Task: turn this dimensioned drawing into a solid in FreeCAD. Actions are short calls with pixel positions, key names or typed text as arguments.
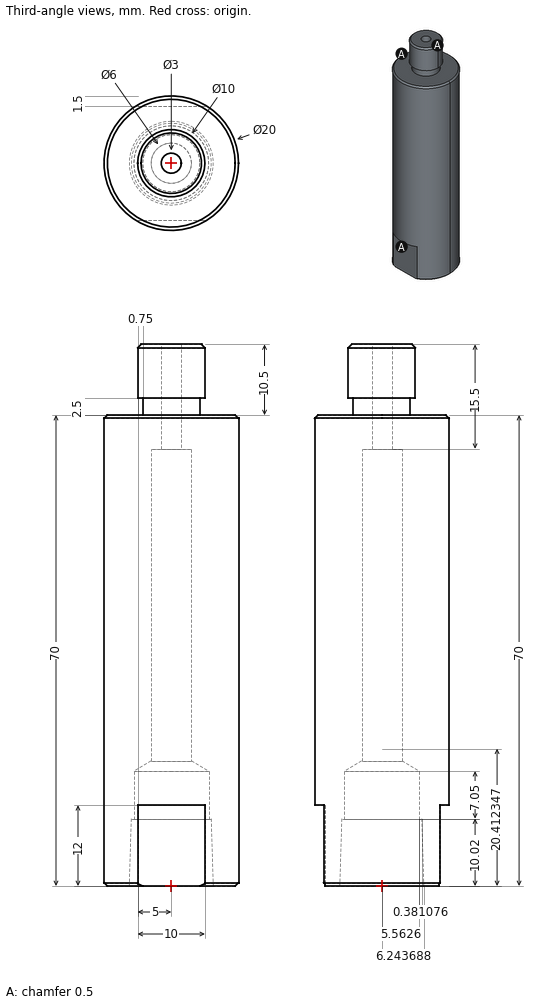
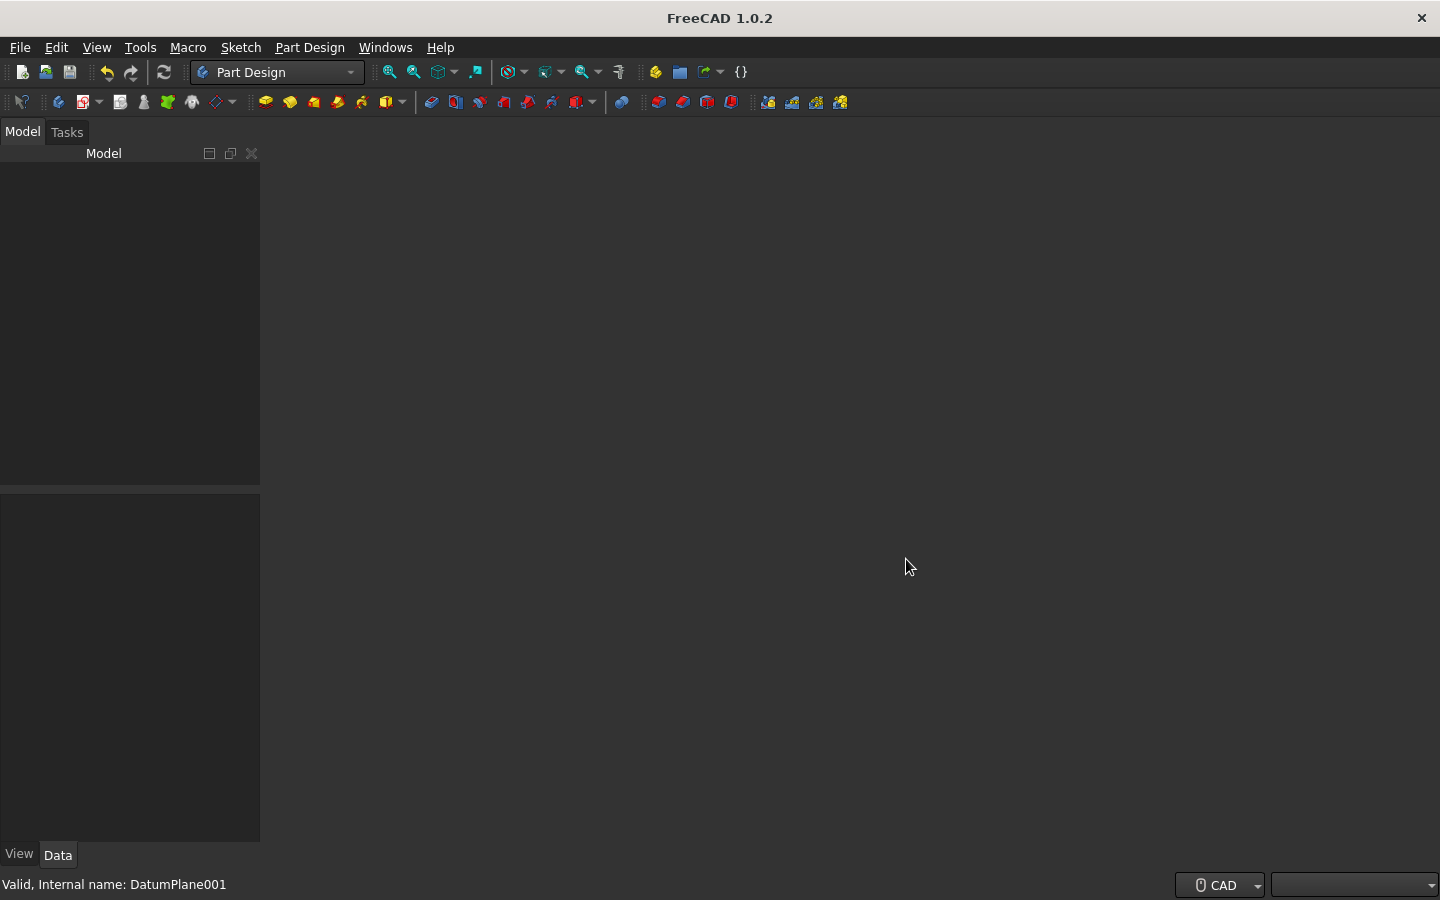
click(22, 72)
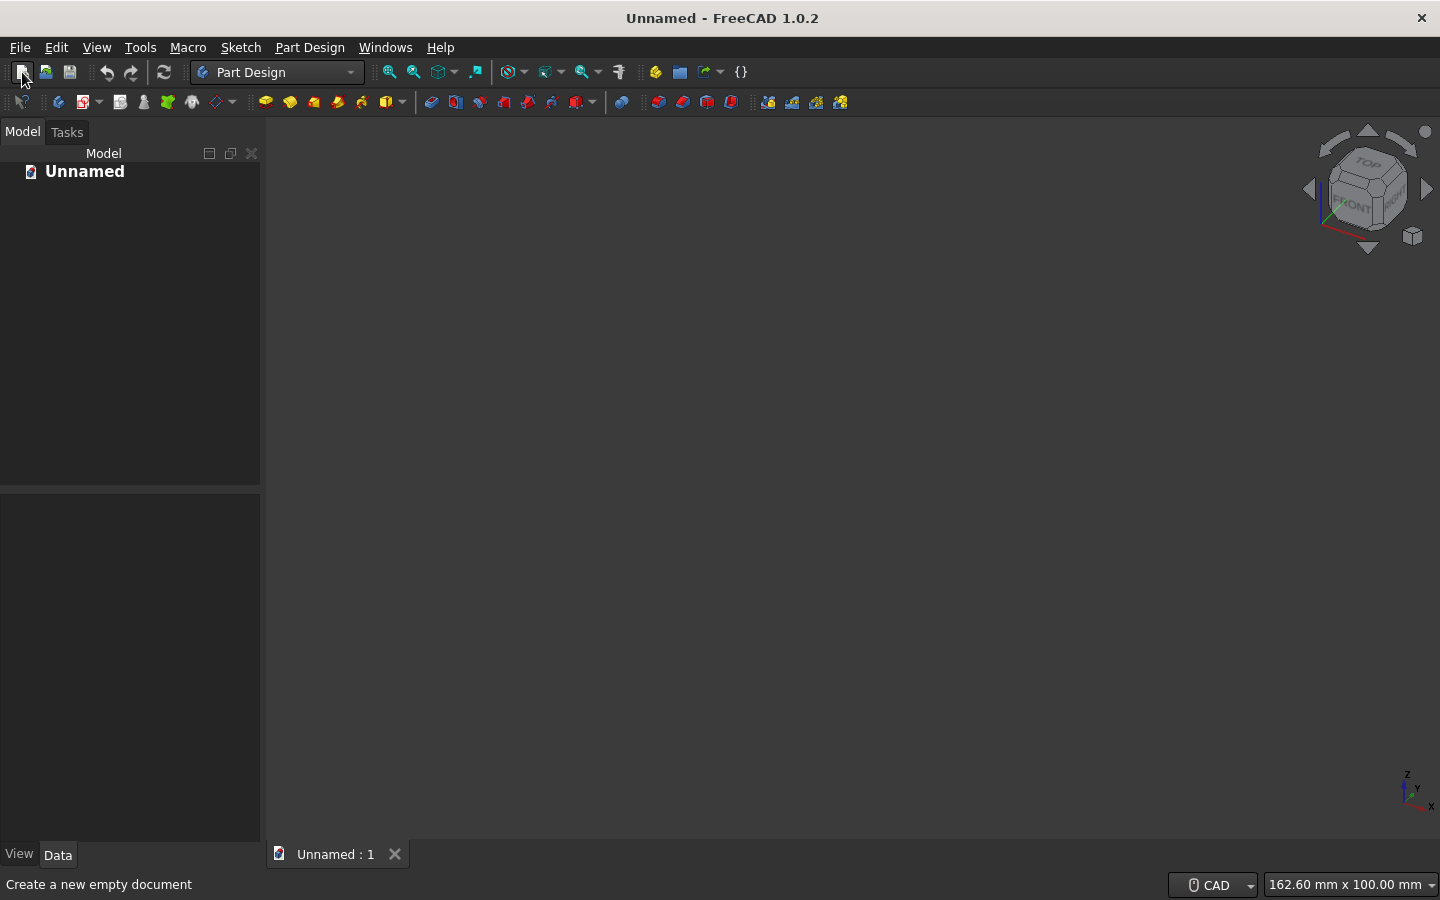
click(84, 102)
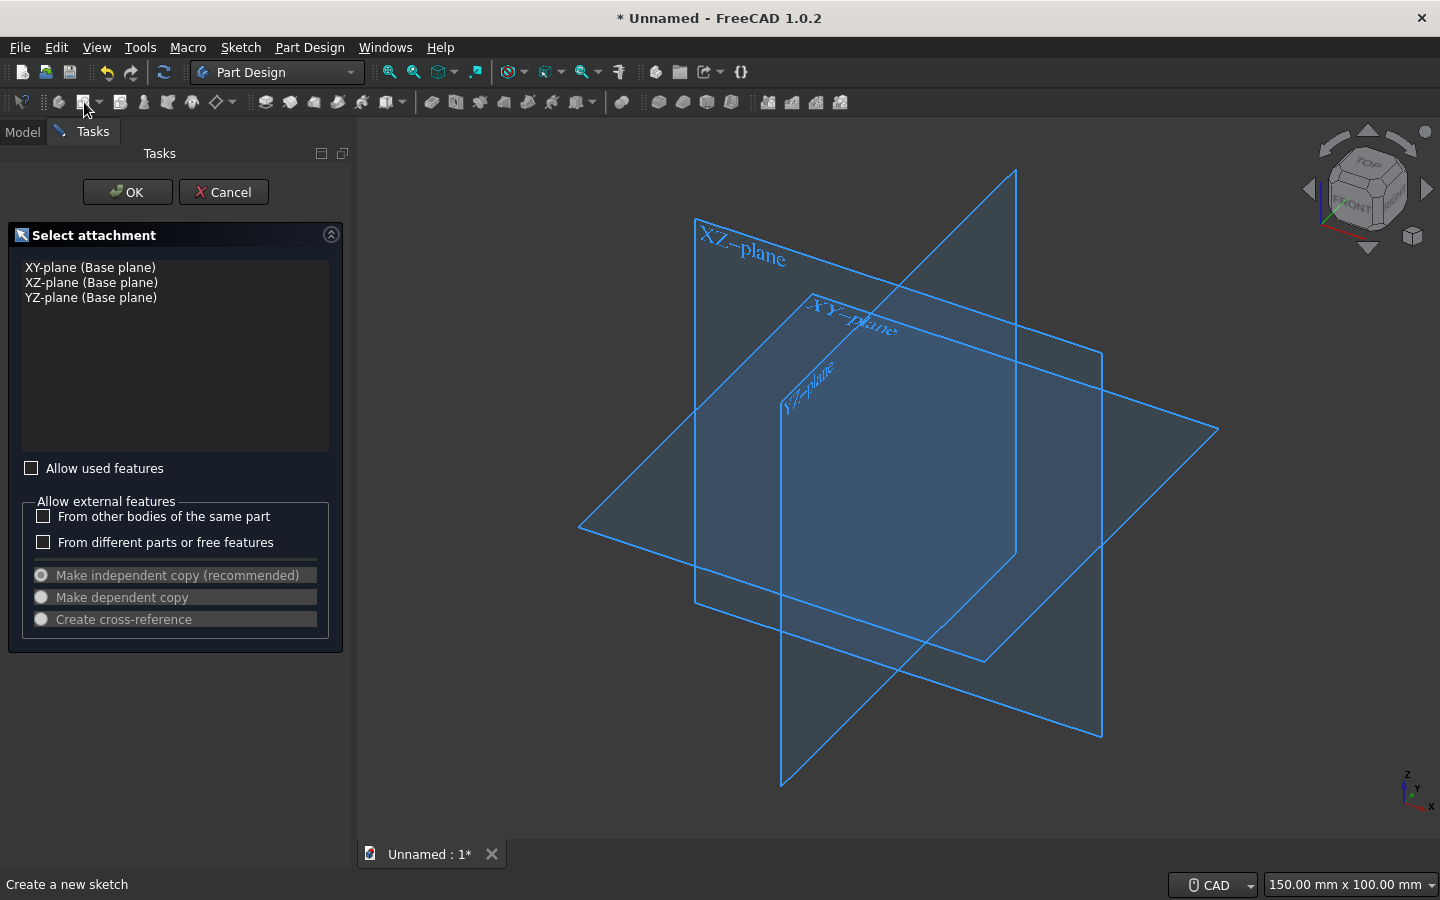
click(82, 268)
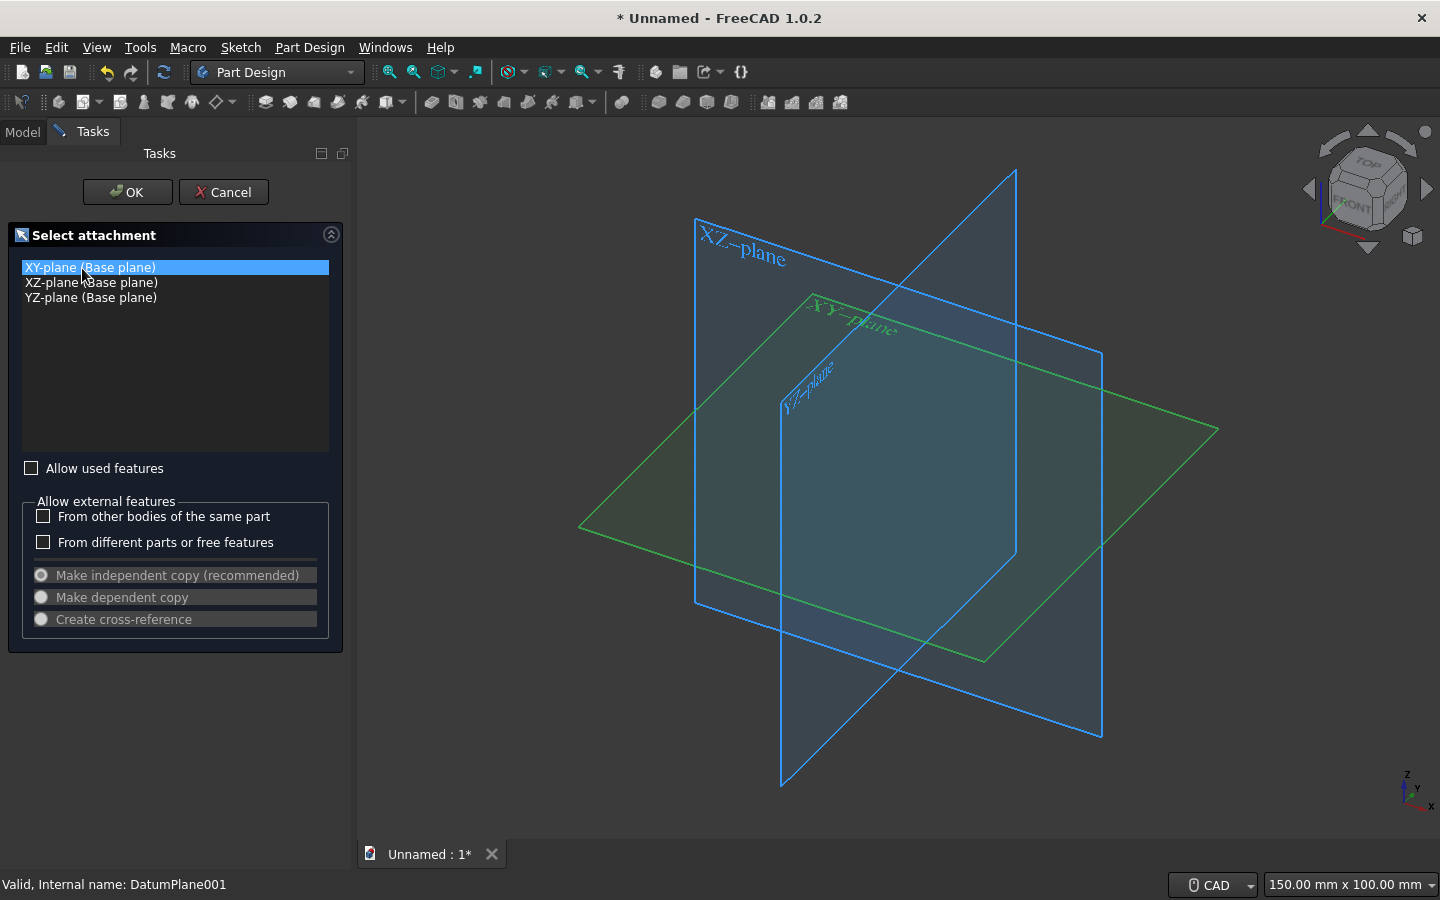
click(128, 192)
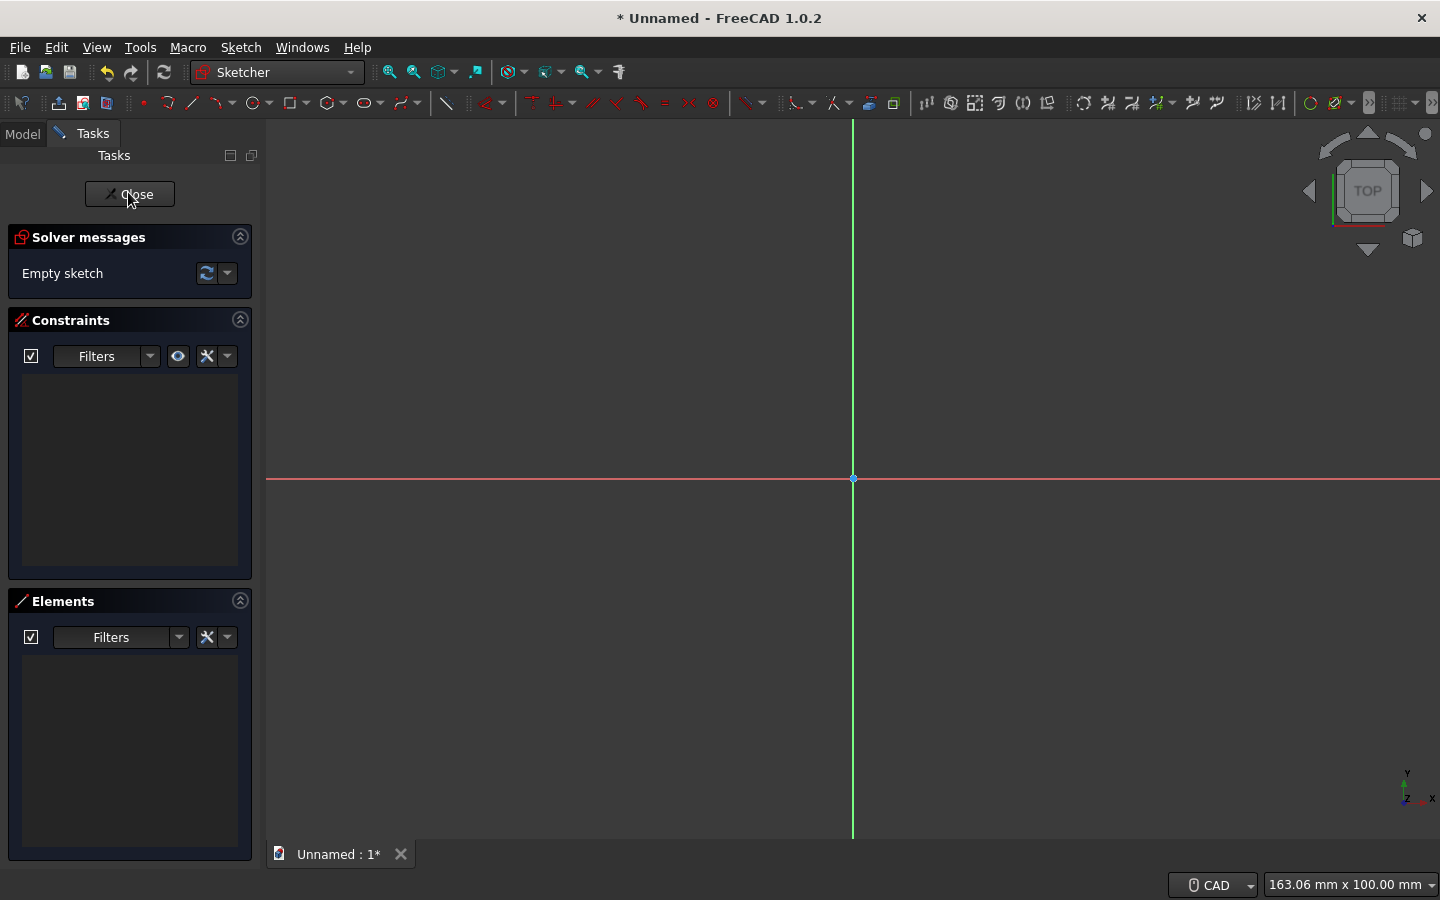
scroll(883, 479, up, 6)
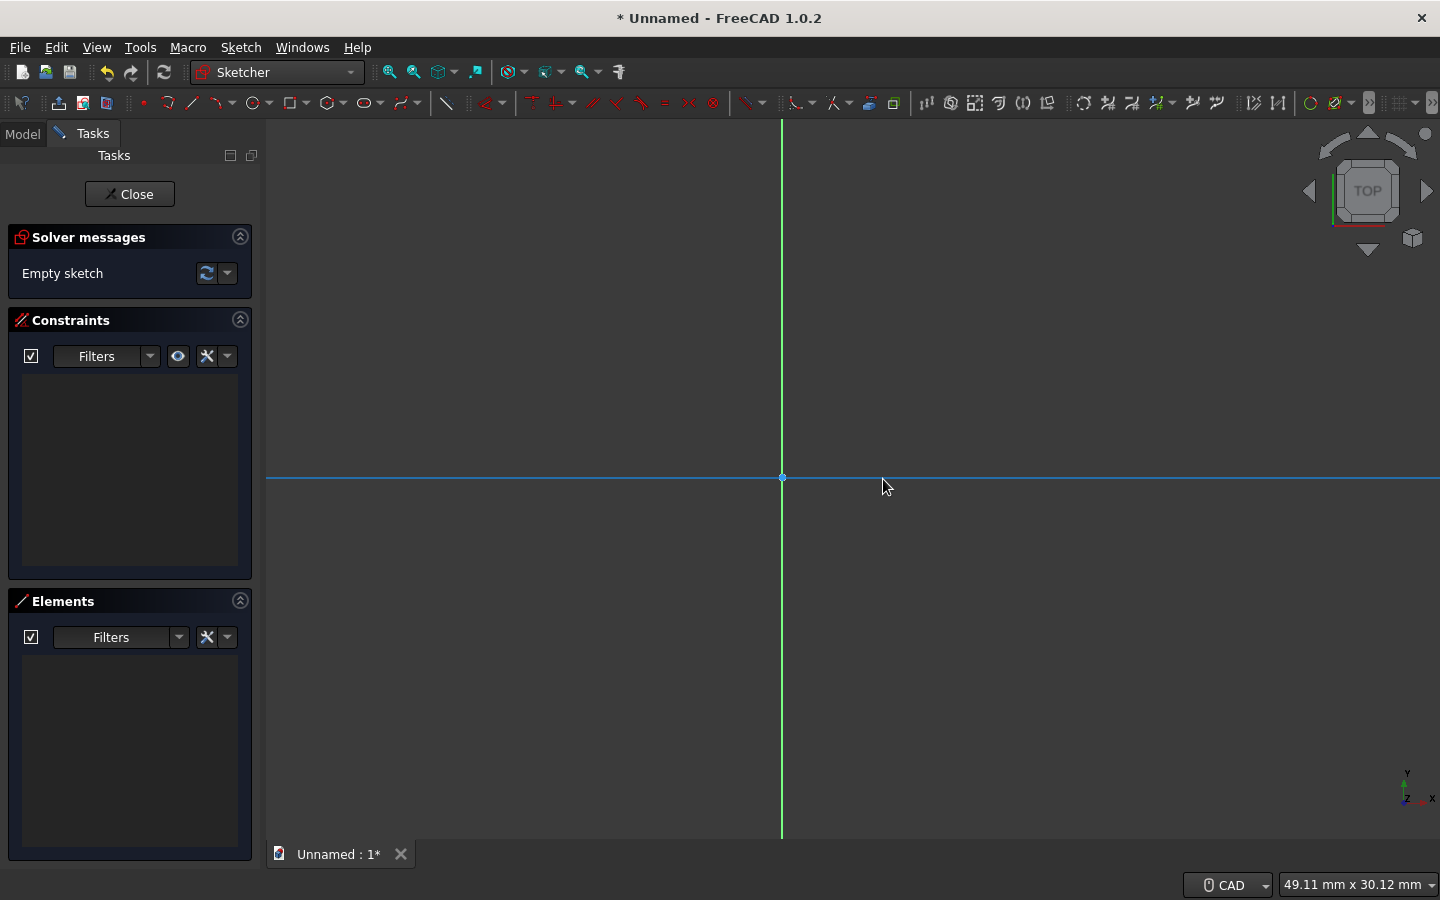
click(254, 104)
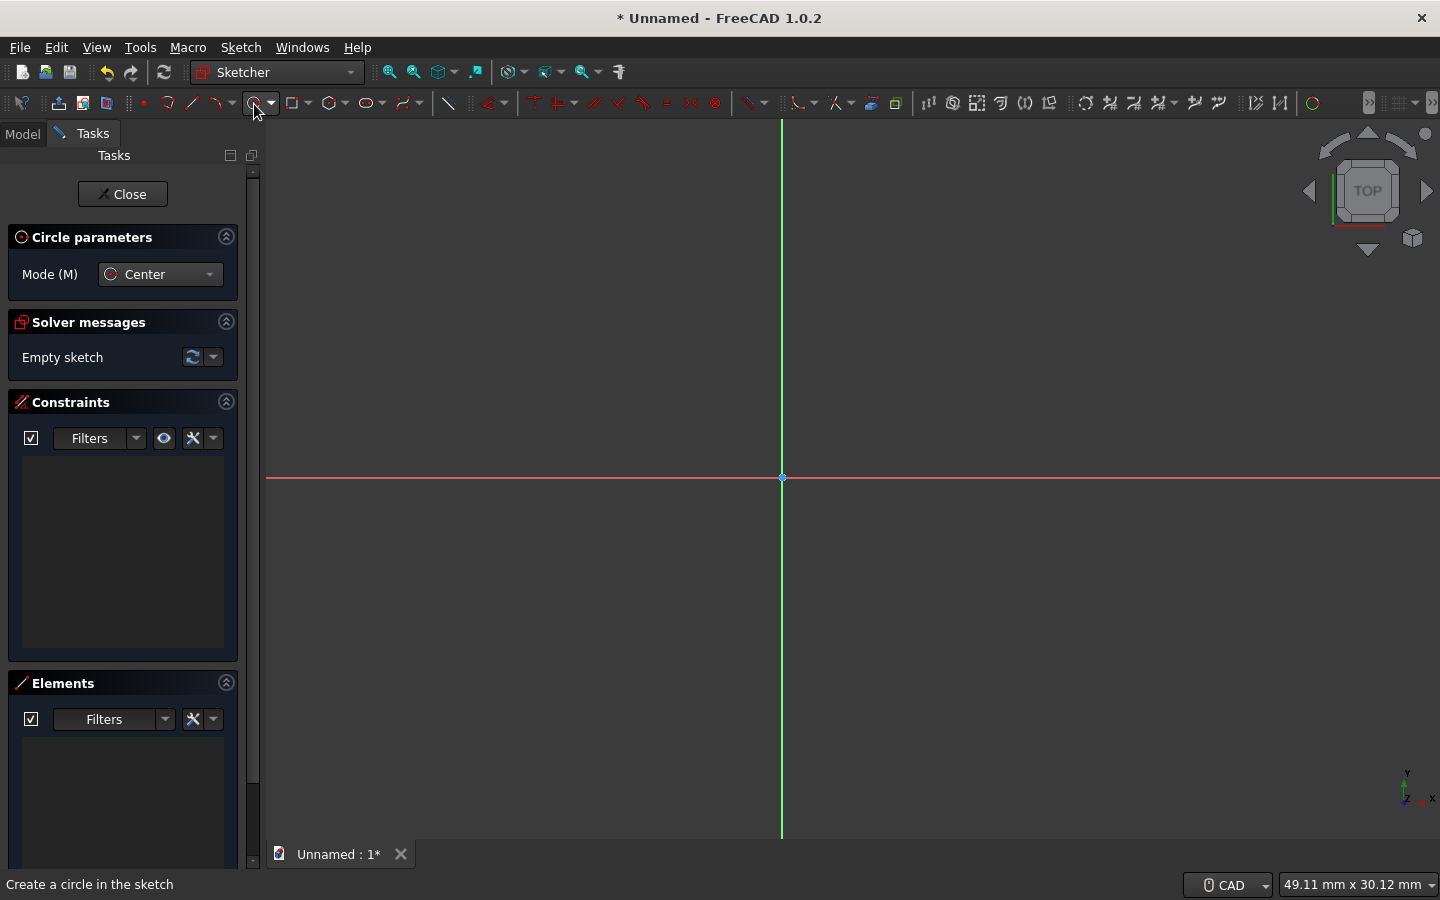
click(782, 478)
move(951, 309)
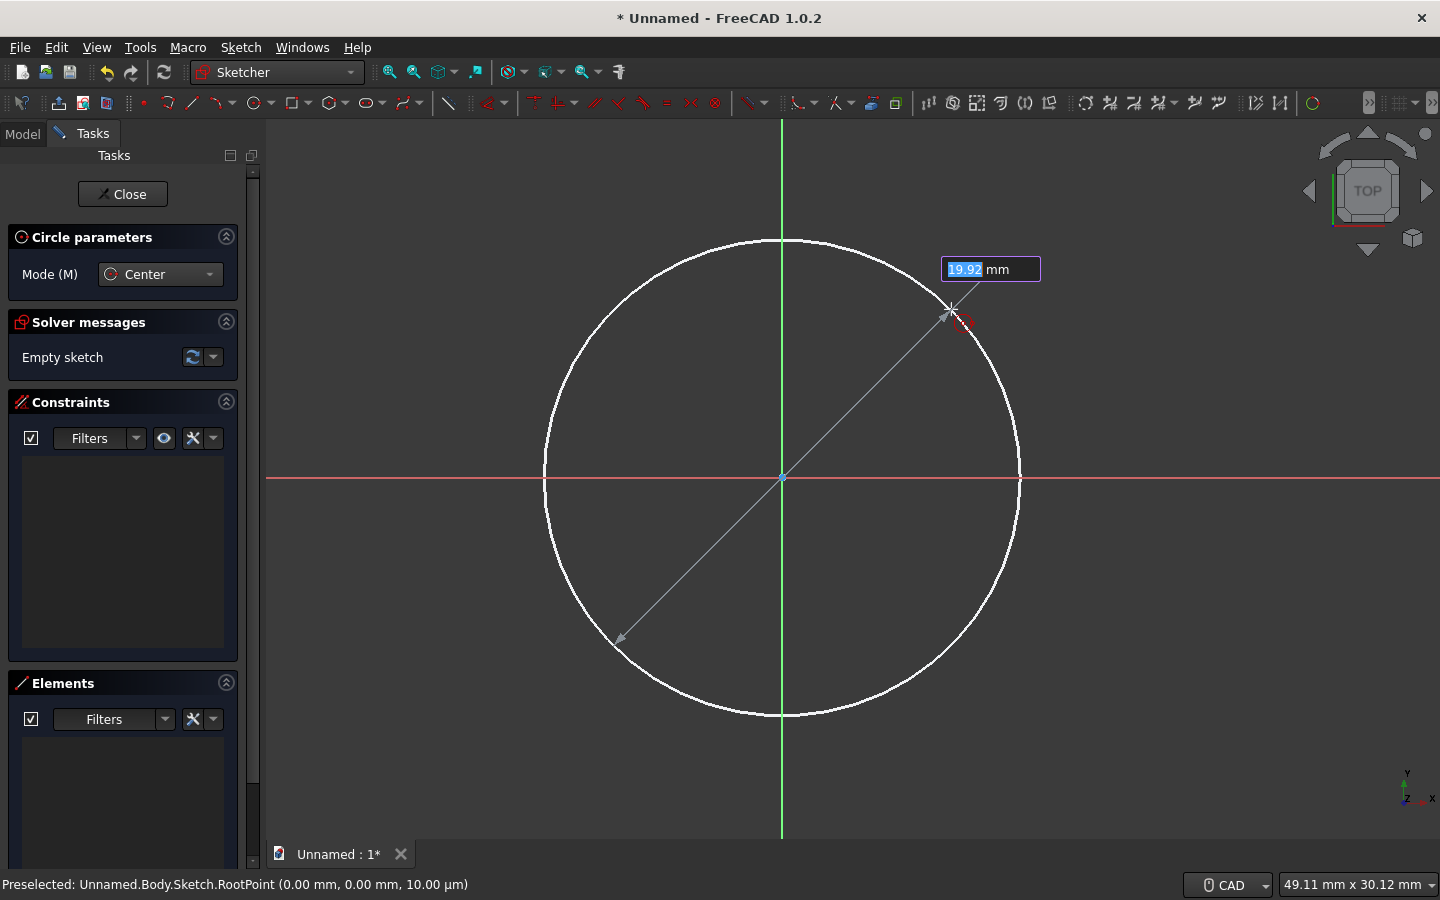
text(20)
key(Return)
key(Escape)